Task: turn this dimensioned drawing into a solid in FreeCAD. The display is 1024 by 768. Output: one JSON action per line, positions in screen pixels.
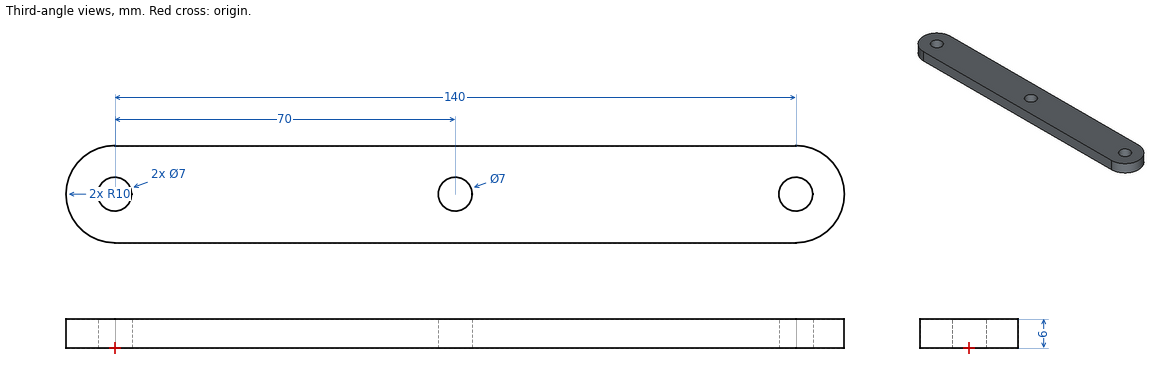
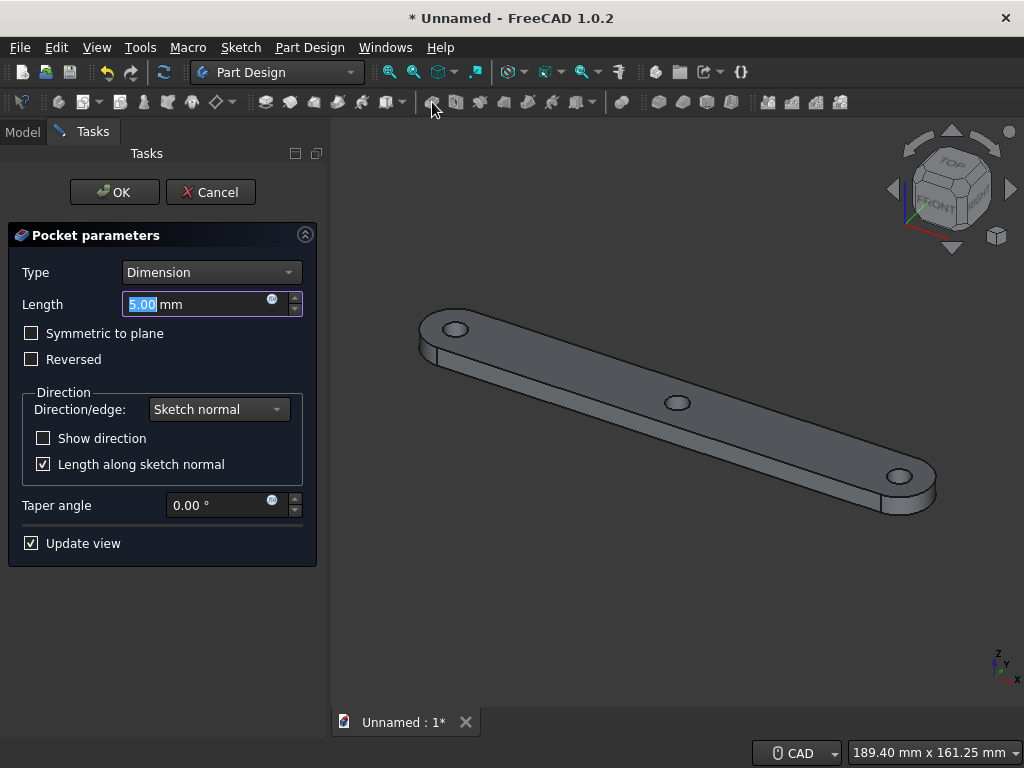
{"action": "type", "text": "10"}
{"action": "key", "text": "Tab"}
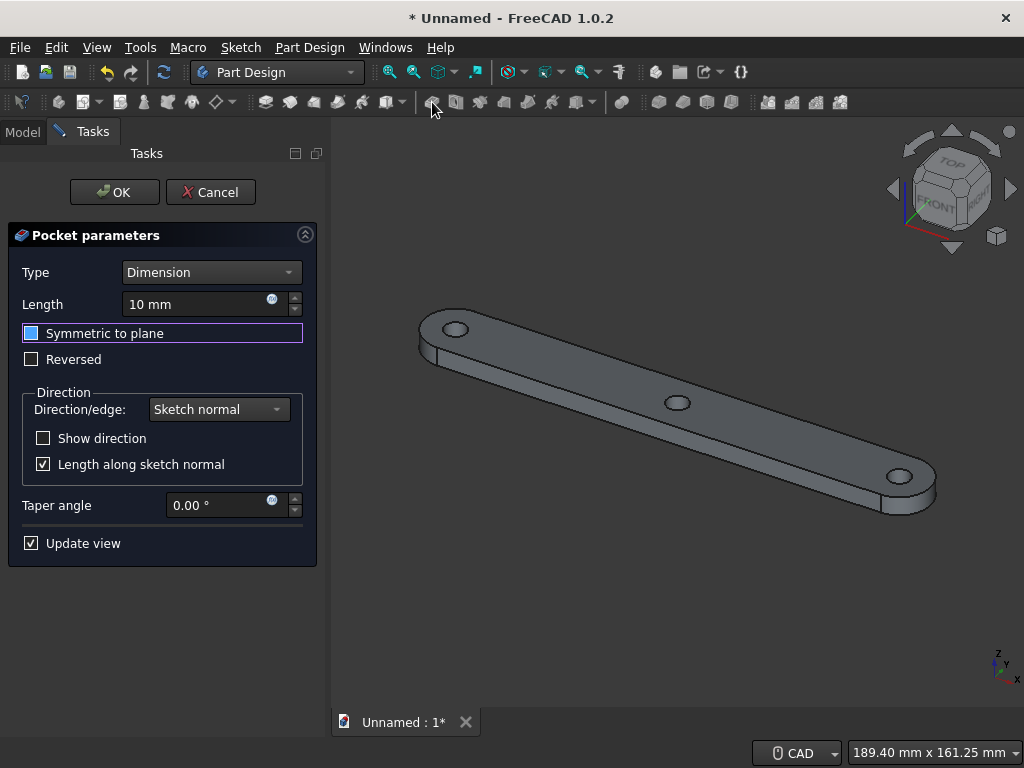
{"action": "left_click", "coordinate": [115, 192]}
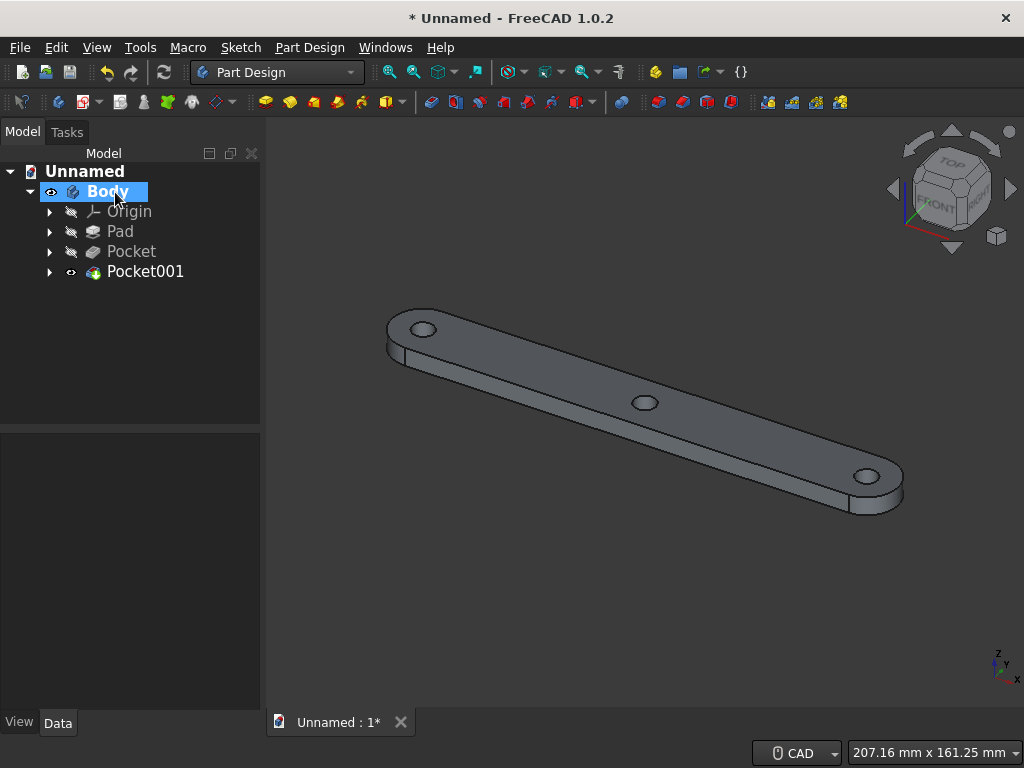
{"action": "key", "text": "0"}